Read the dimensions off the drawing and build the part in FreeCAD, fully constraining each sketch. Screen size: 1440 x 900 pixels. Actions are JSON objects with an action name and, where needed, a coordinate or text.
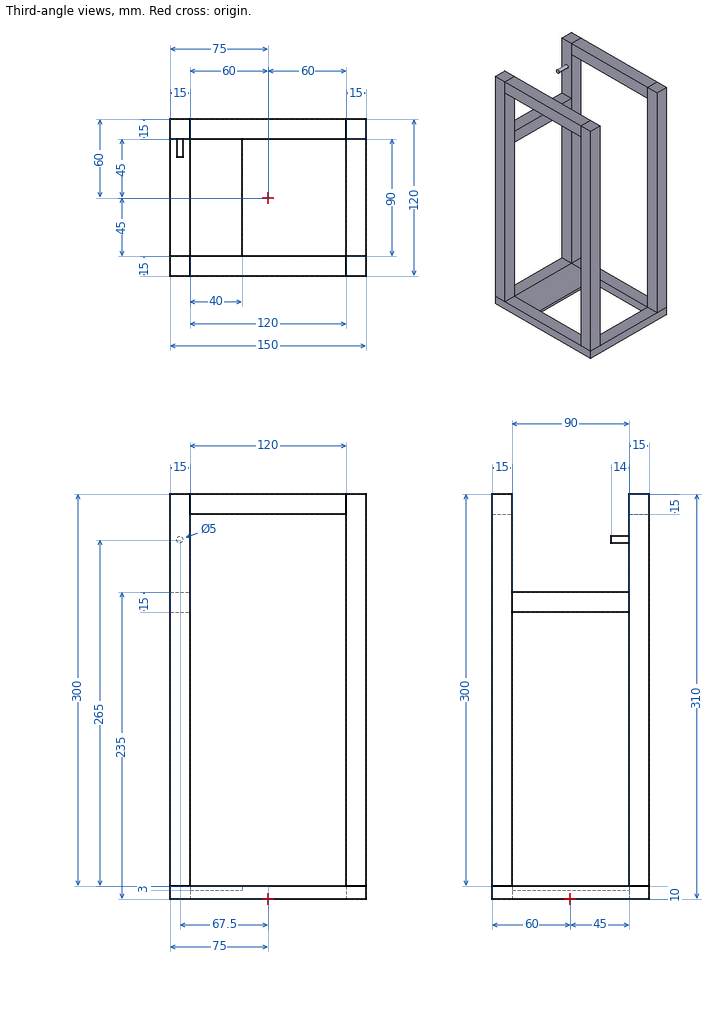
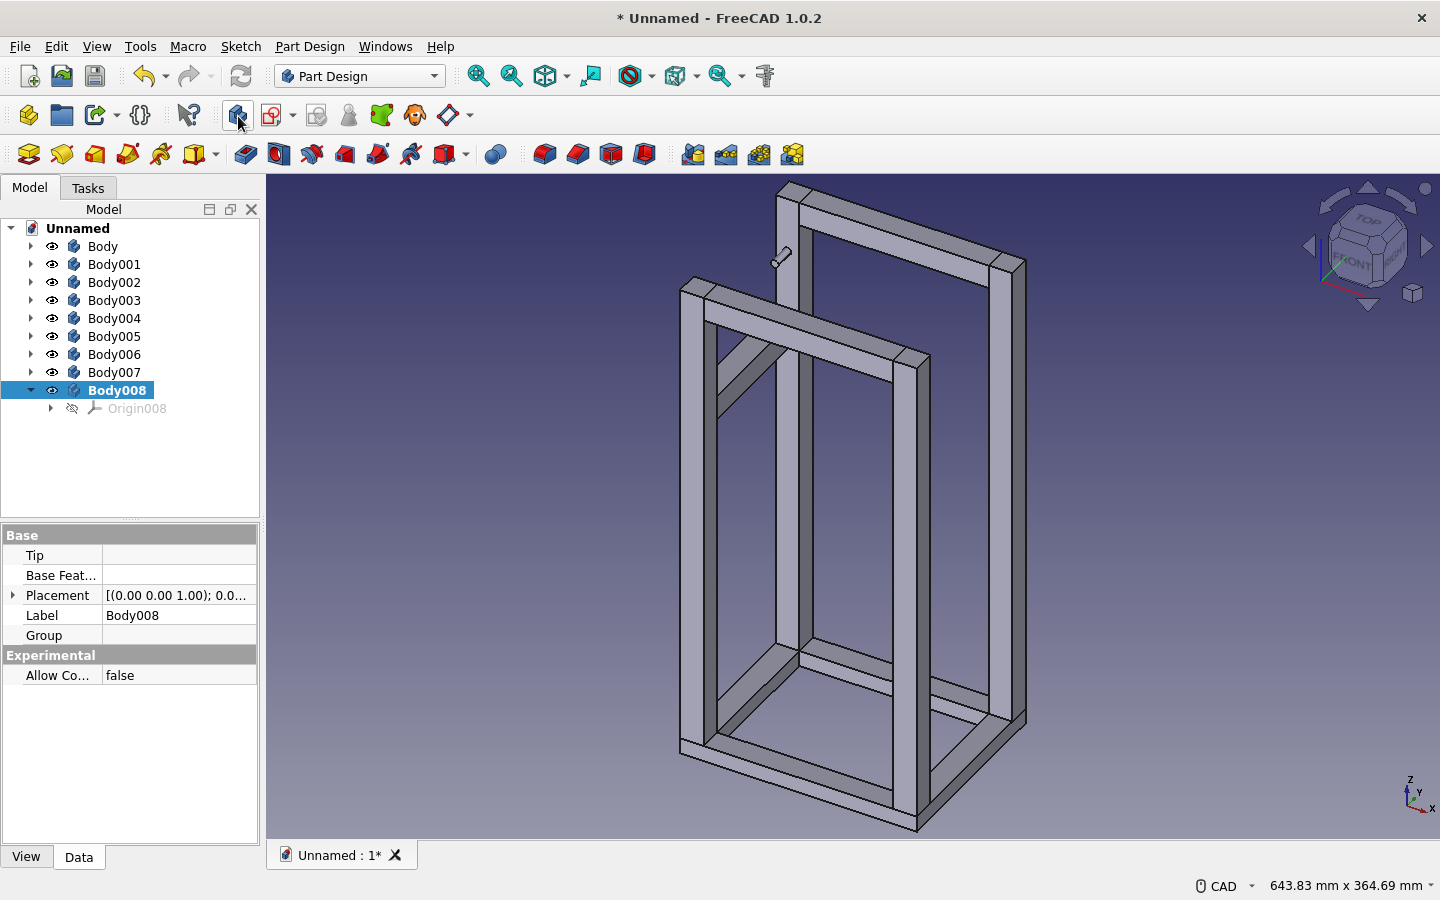
{"action": "left_click", "coordinate": [51, 408]}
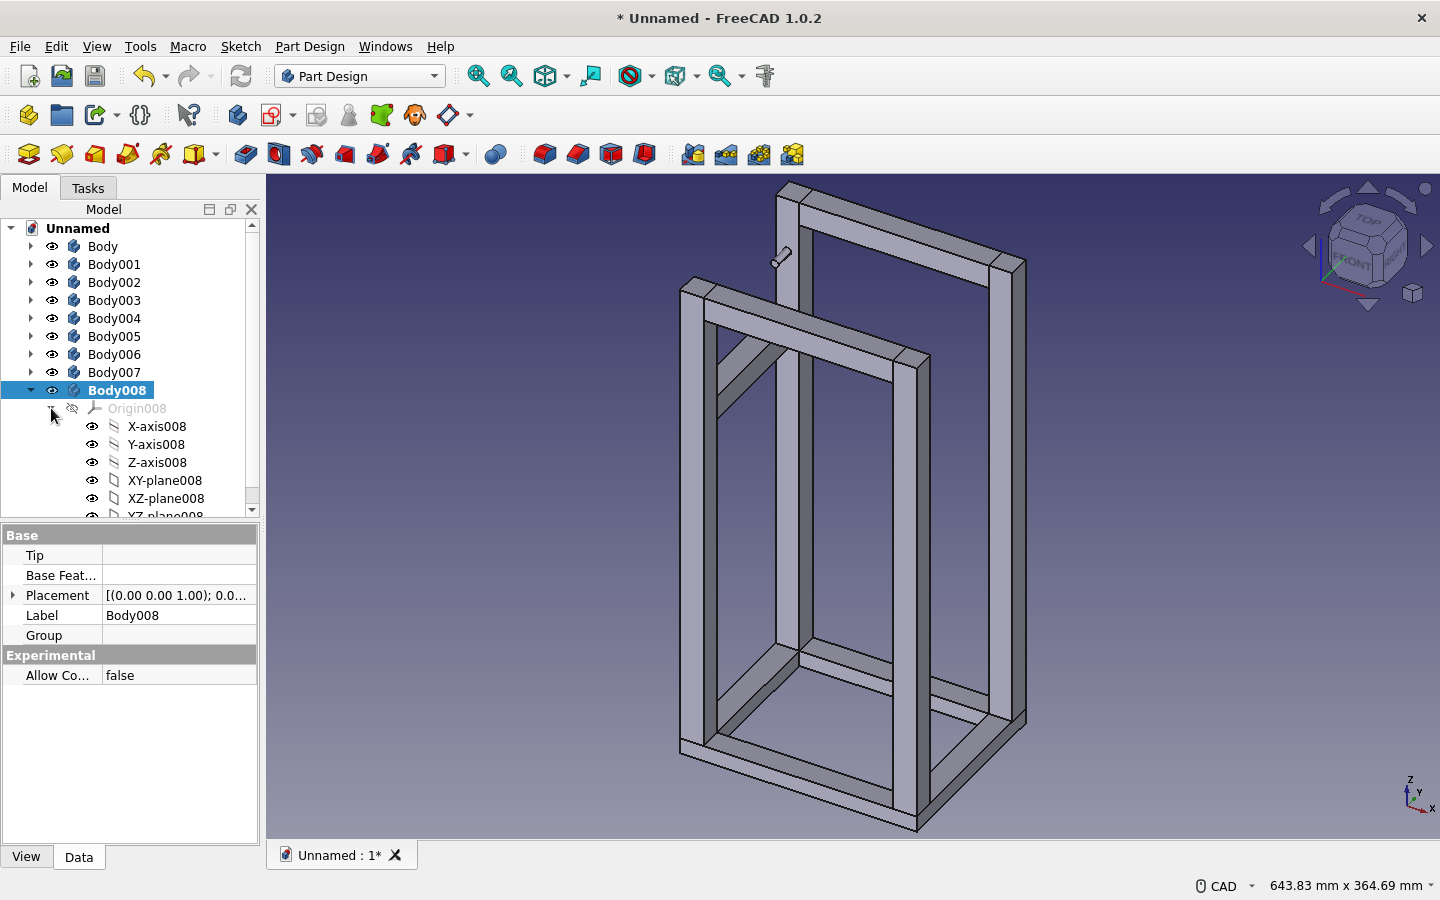
{"action": "left_click", "coordinate": [137, 480]}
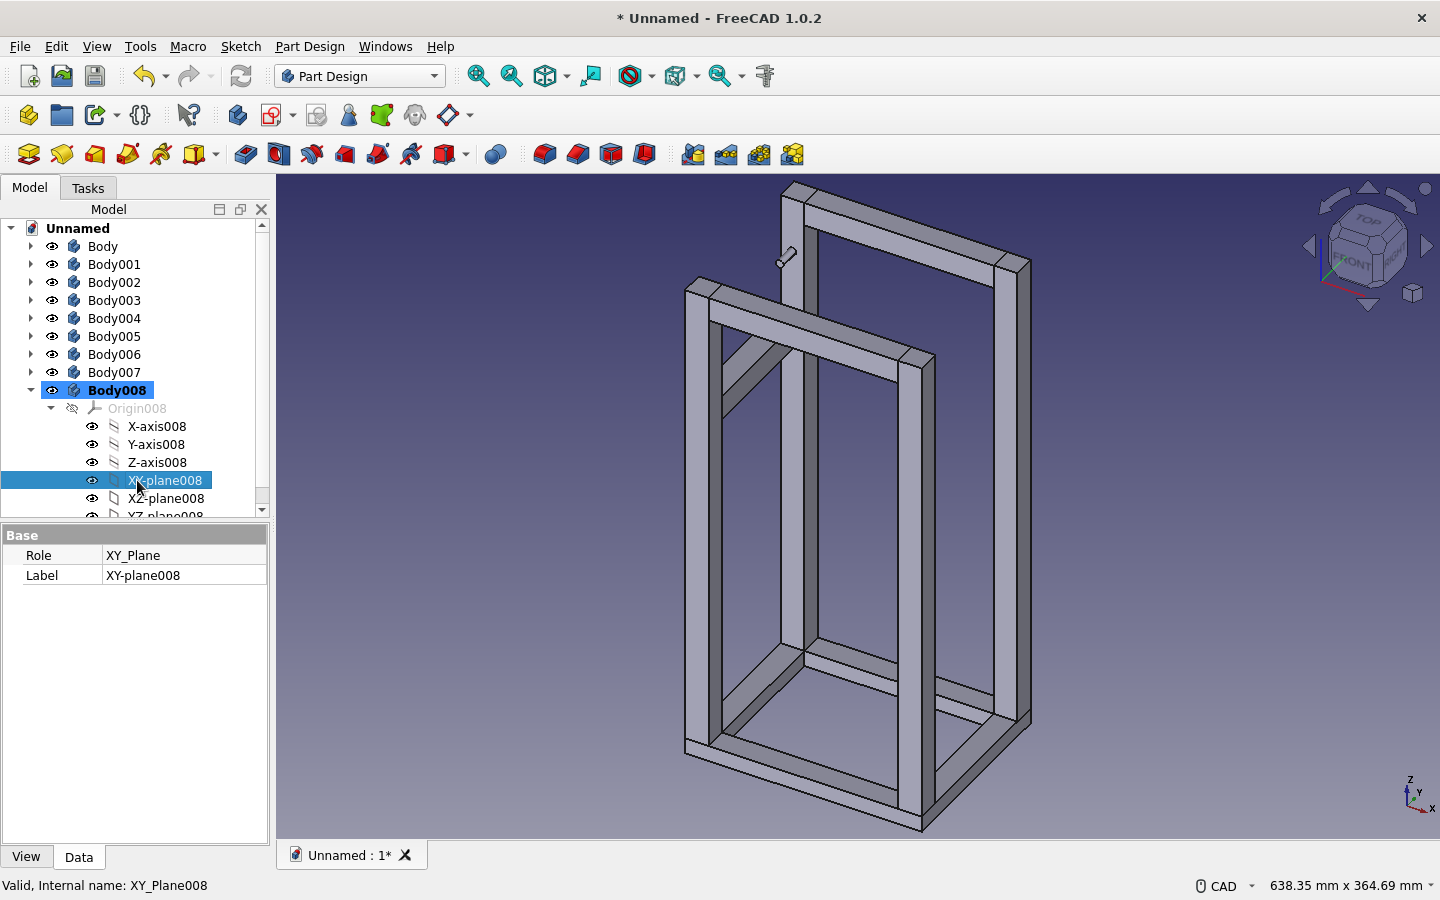
{"action": "left_click", "coordinate": [448, 116]}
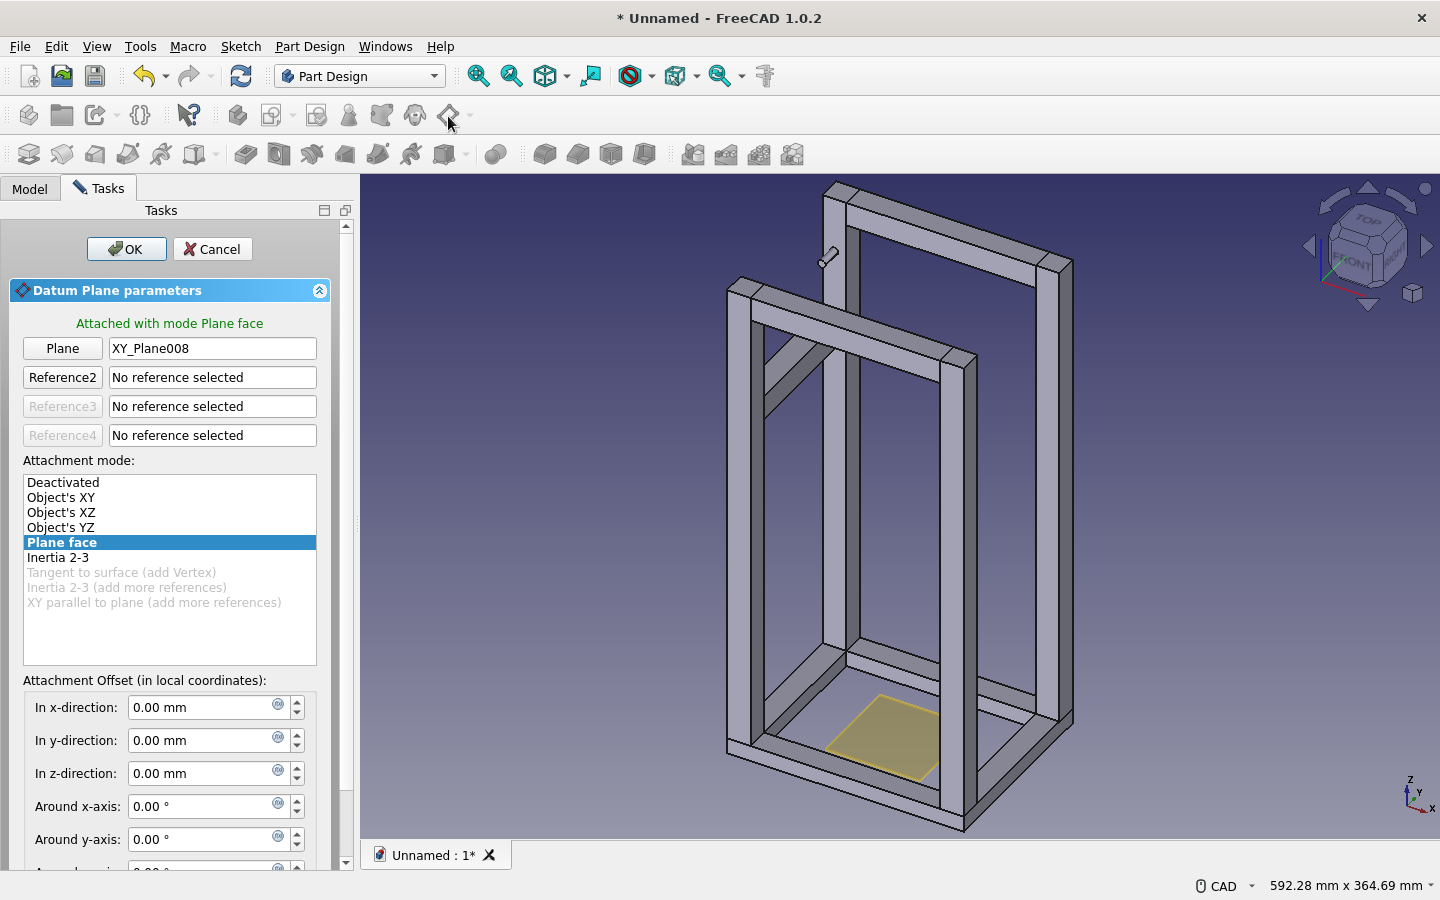
{"action": "triple_click", "coordinate": [210, 774]}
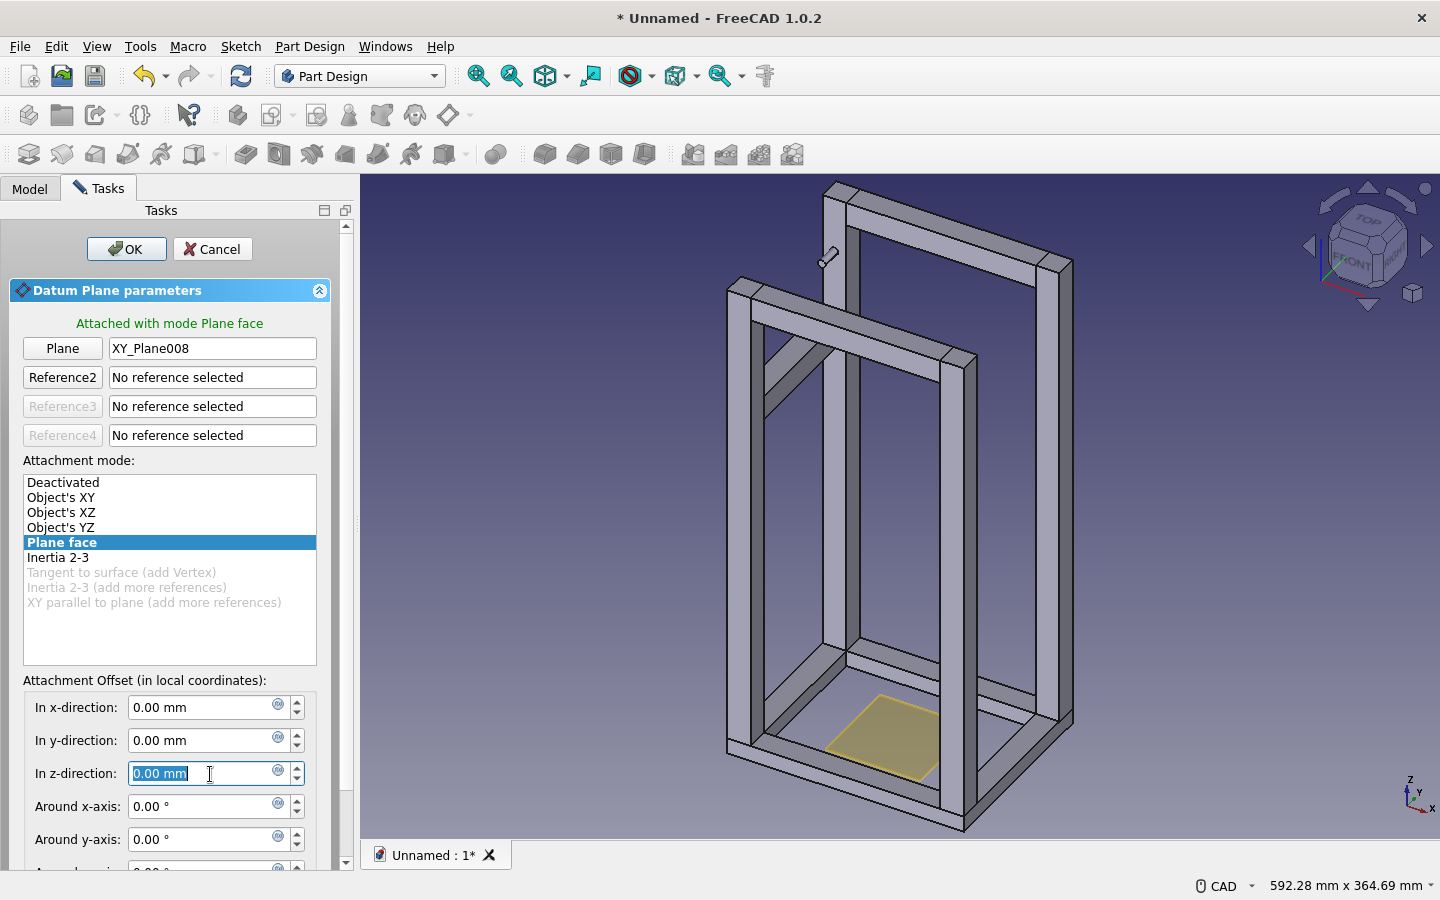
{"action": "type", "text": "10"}
{"action": "key", "text": "Tab"}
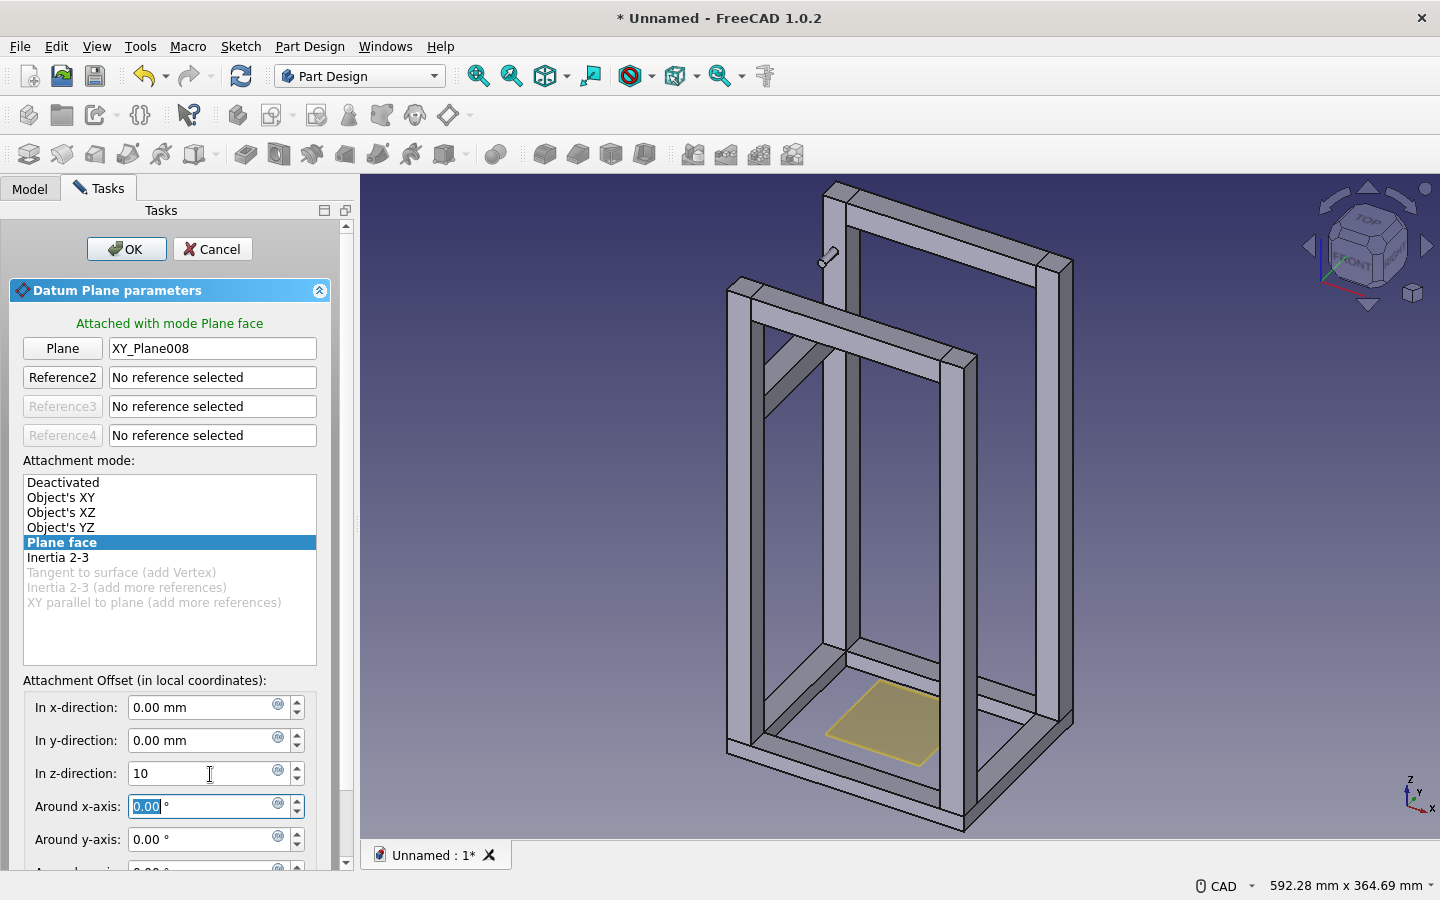
{"action": "left_click", "coordinate": [127, 249]}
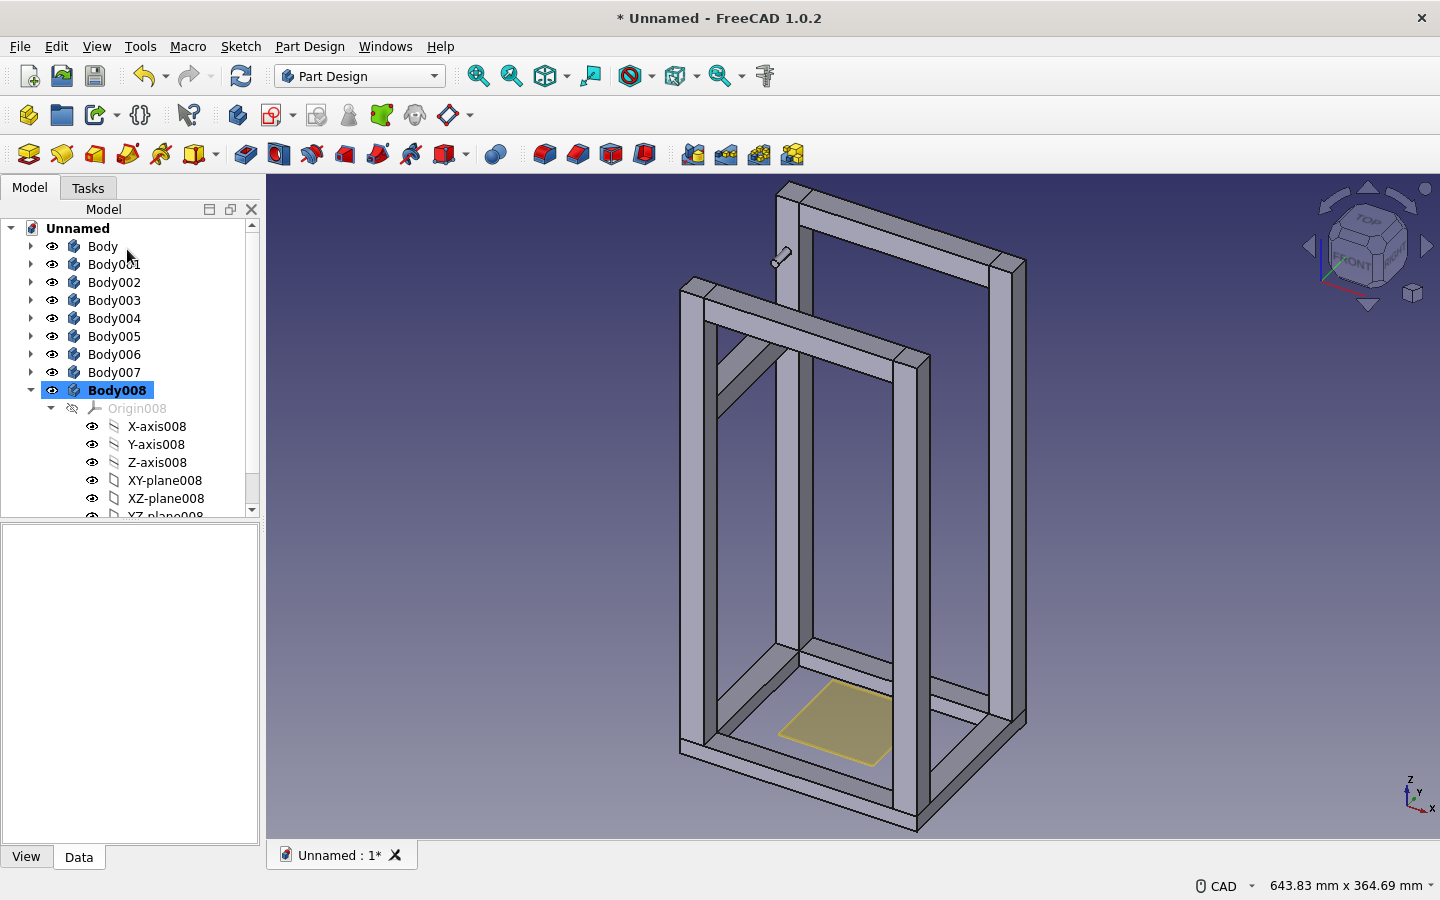
{"action": "scroll", "coordinate": [101, 368], "scroll_direction": "down", "scroll_amount": 3}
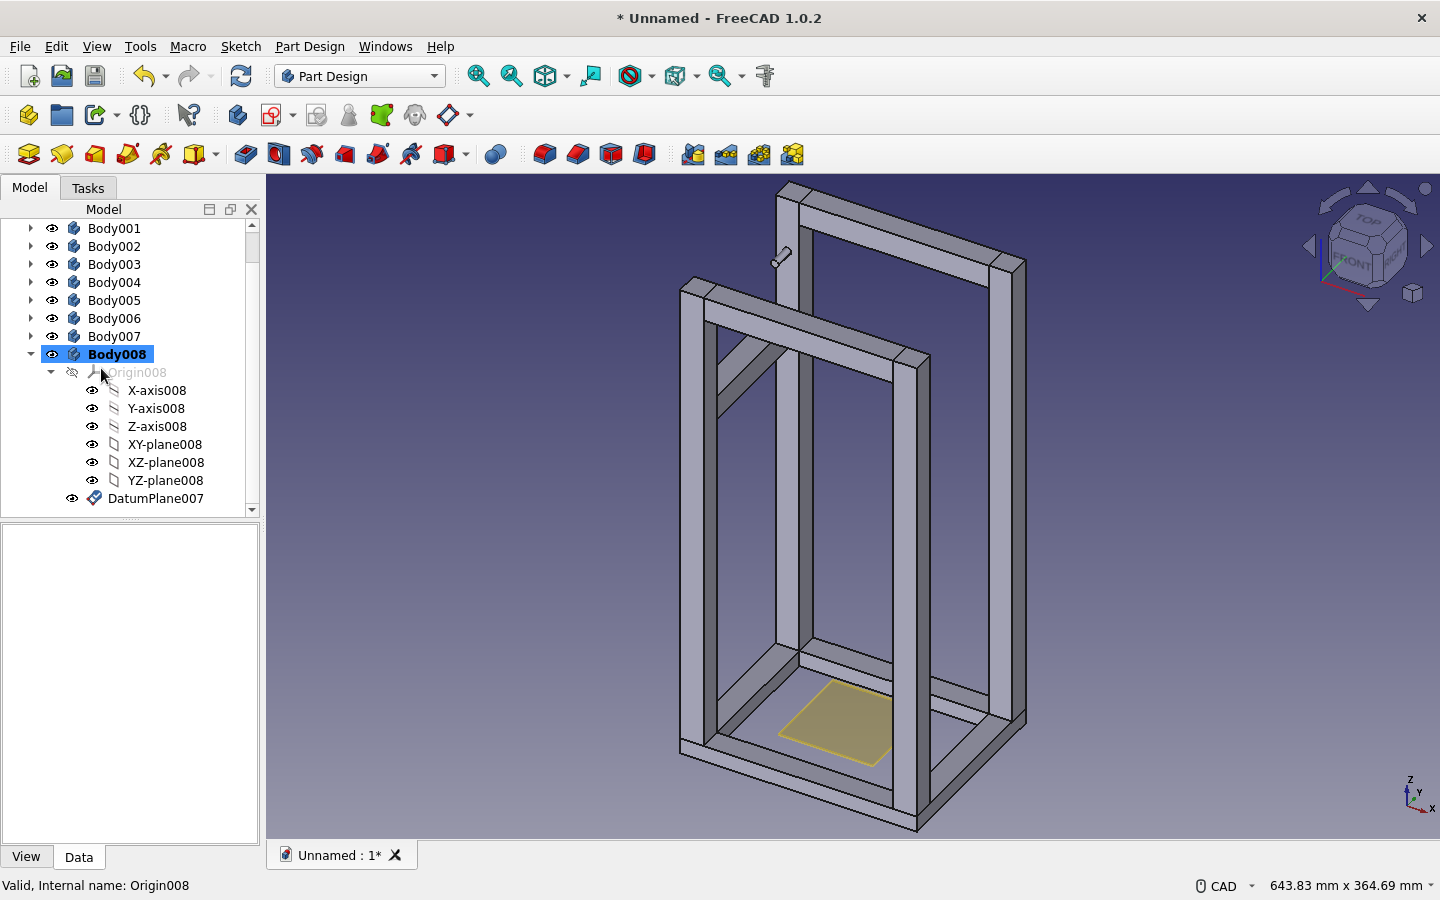
{"action": "left_click", "coordinate": [117, 498]}